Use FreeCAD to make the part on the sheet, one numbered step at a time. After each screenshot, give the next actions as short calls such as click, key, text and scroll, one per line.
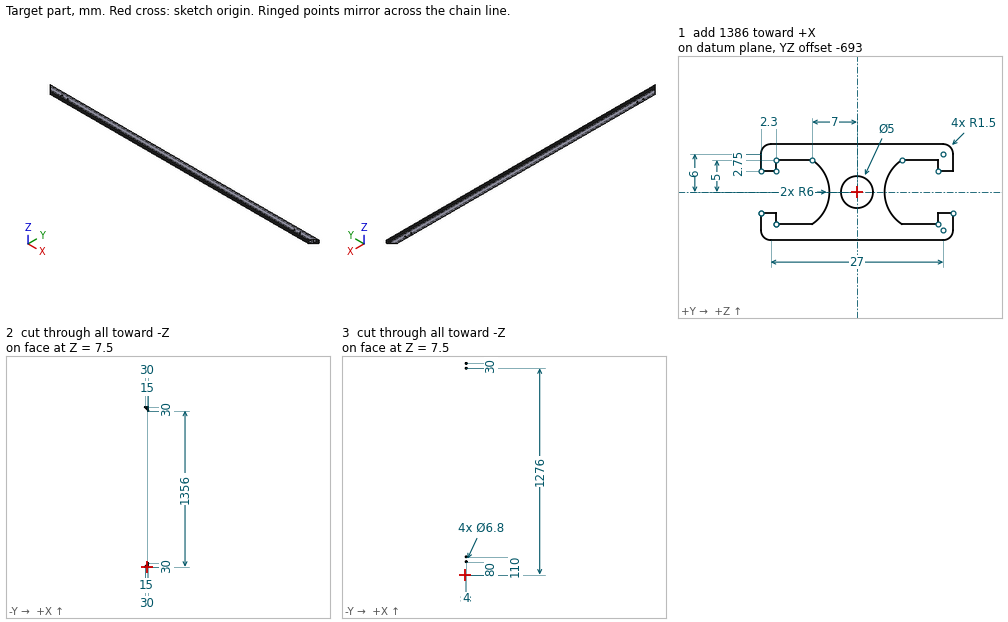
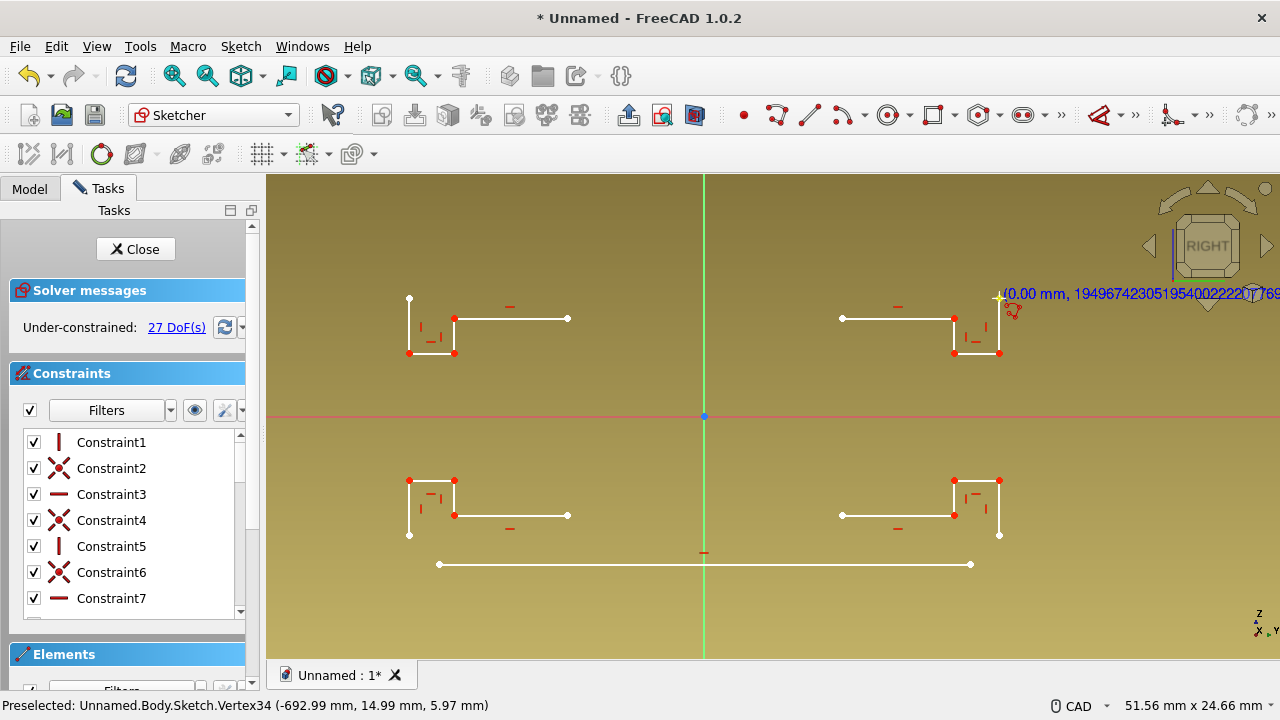
click(810, 116)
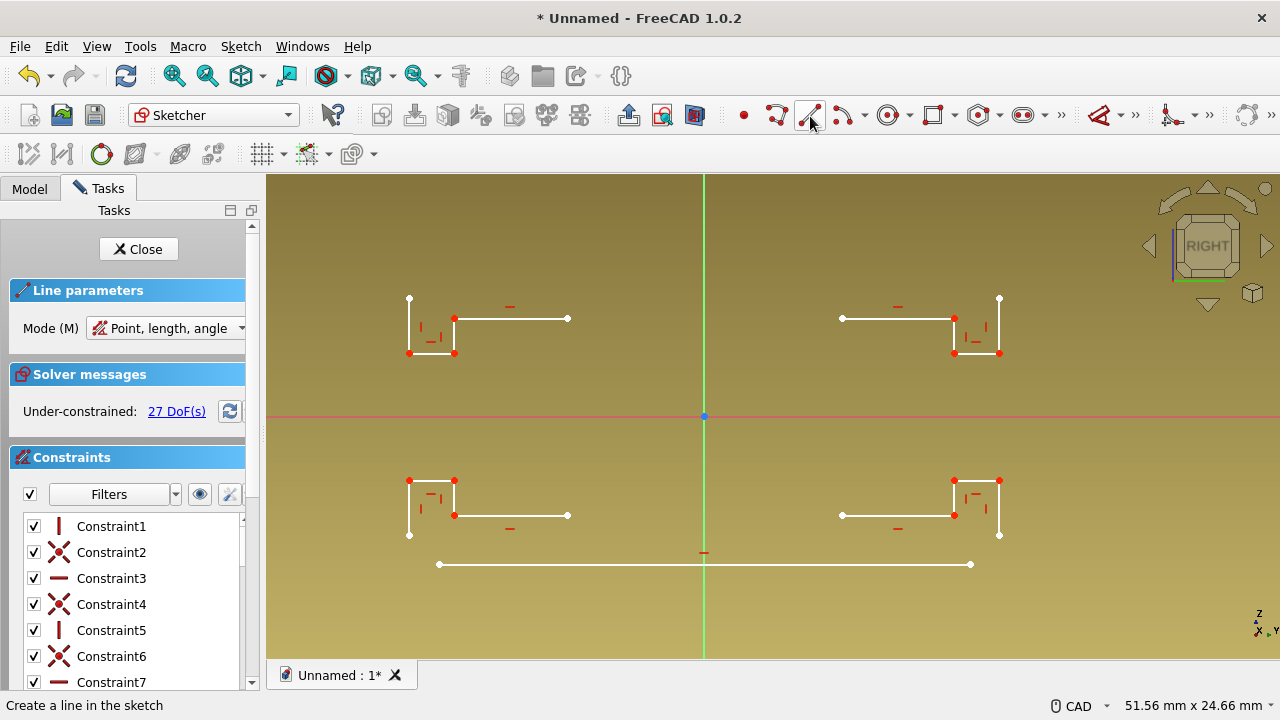
click(970, 269)
click(439, 269)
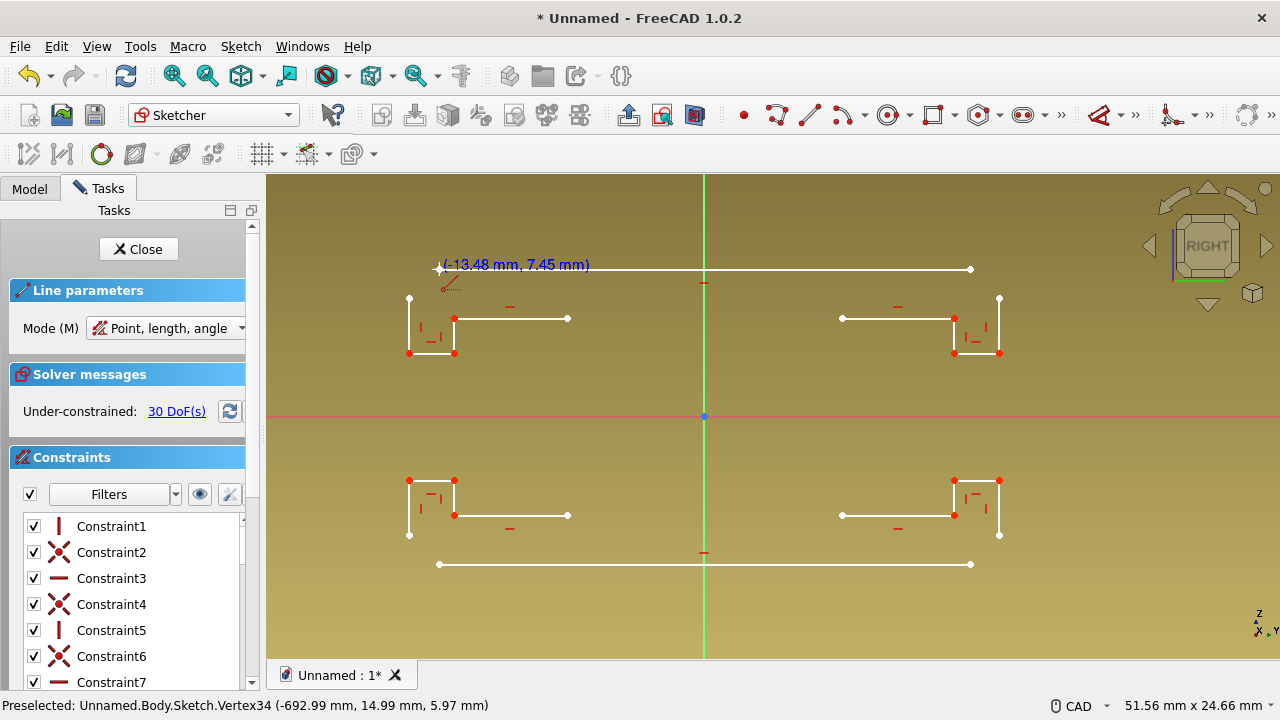
click(864, 116)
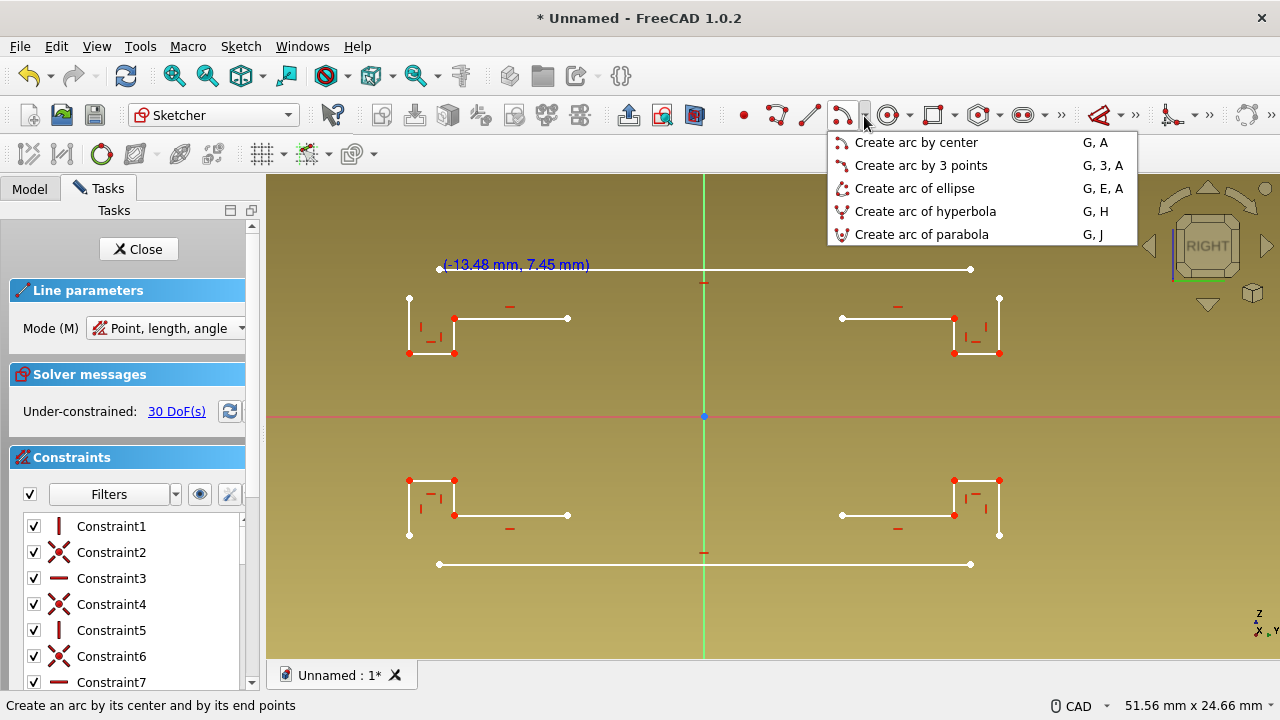
click(982, 166)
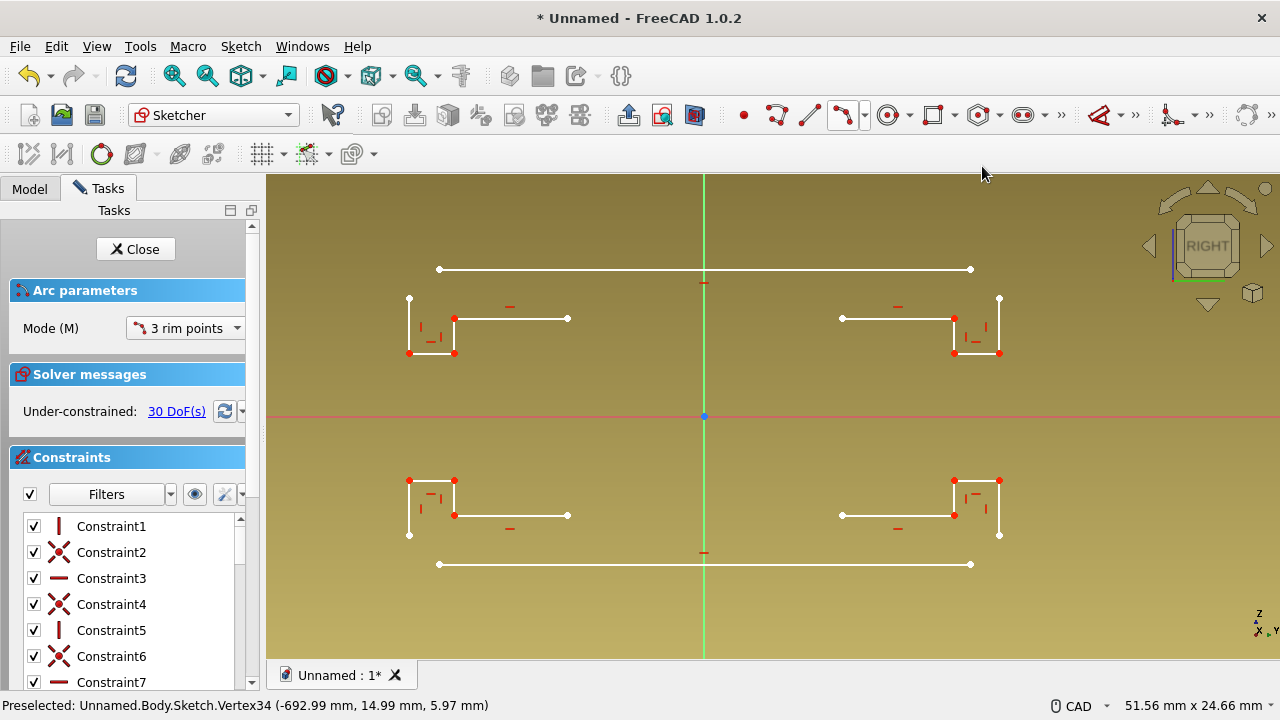
click(567, 319)
click(567, 516)
click(617, 440)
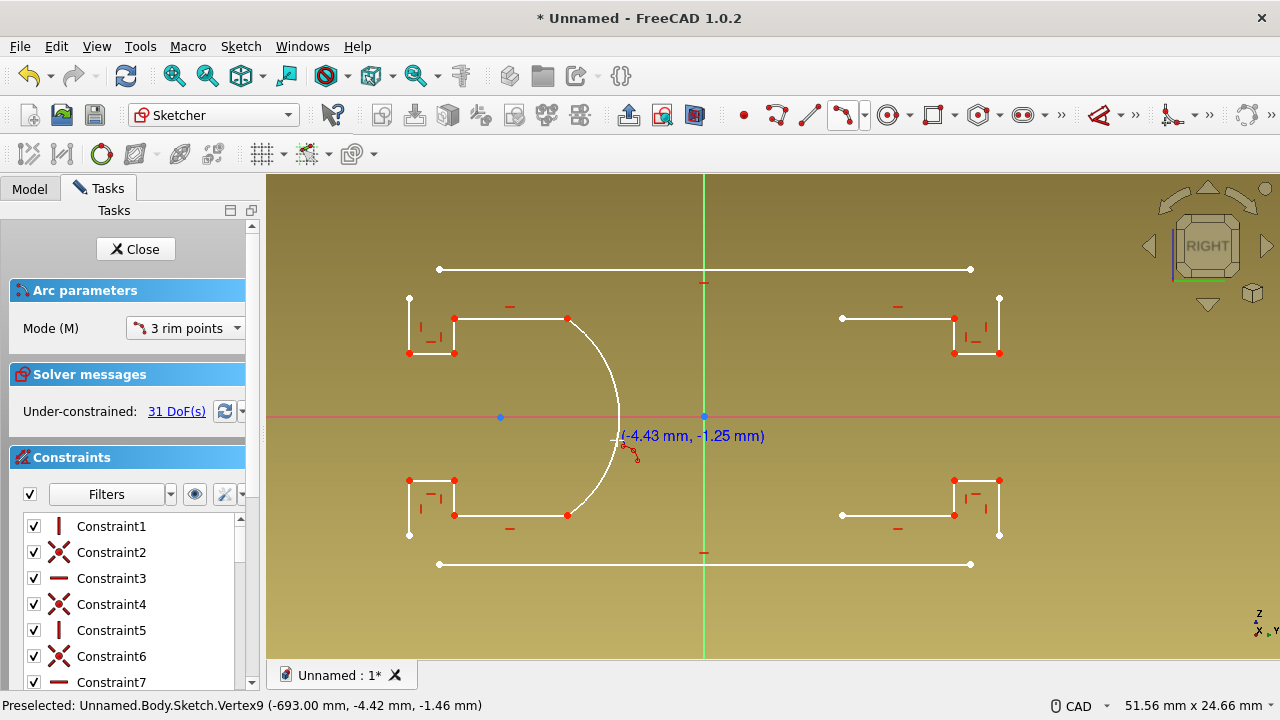
click(409, 536)
click(439, 565)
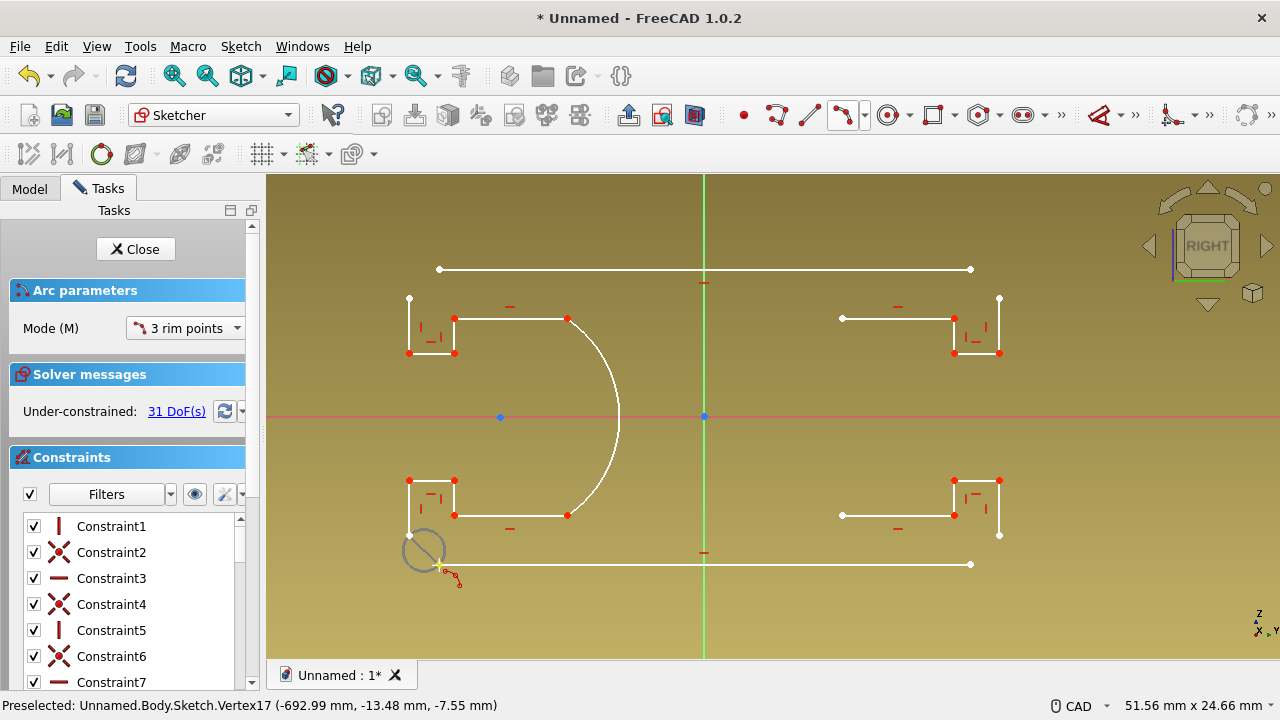
scroll(418, 555, up, 4)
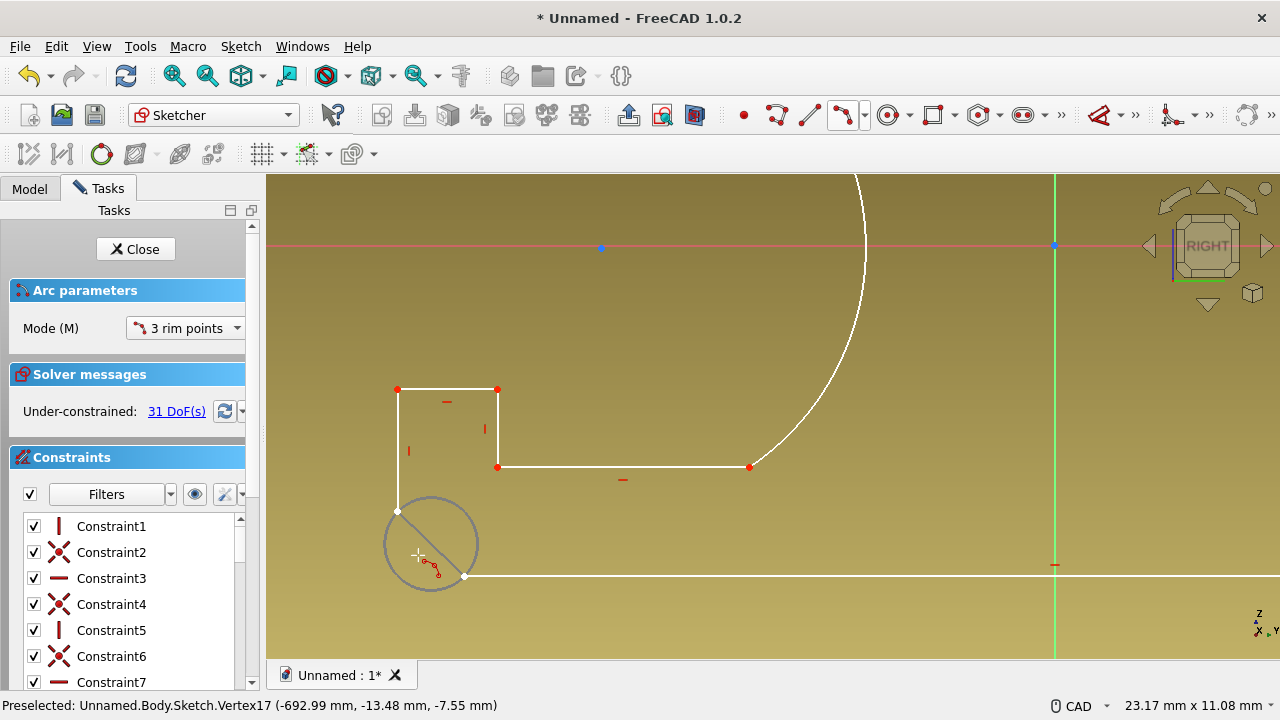
click(417, 555)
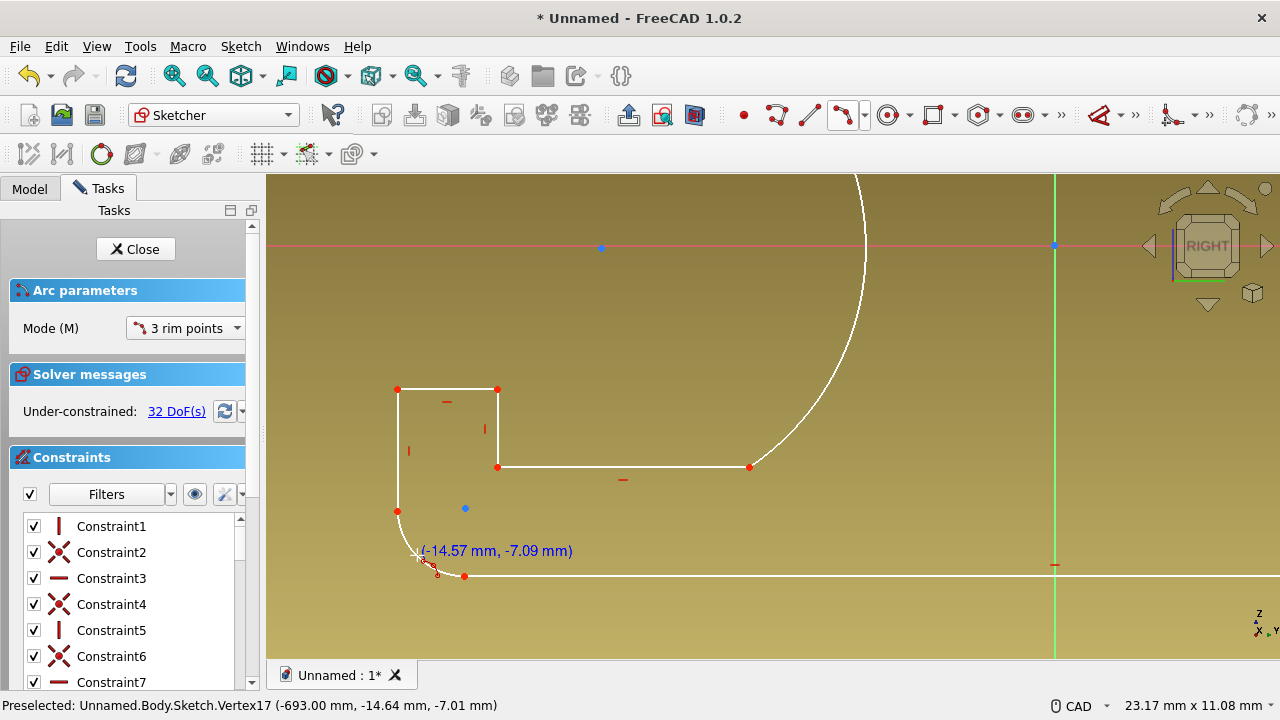
scroll(419, 556, down, 4)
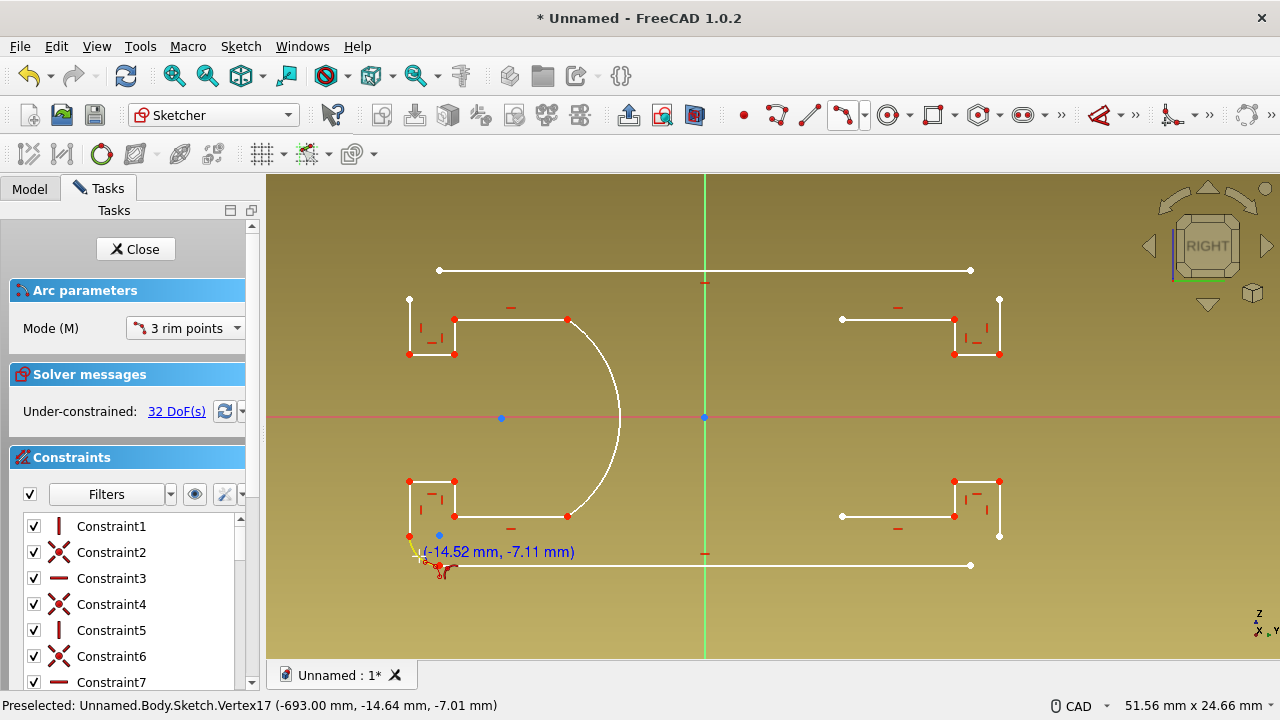
click(971, 566)
click(1000, 537)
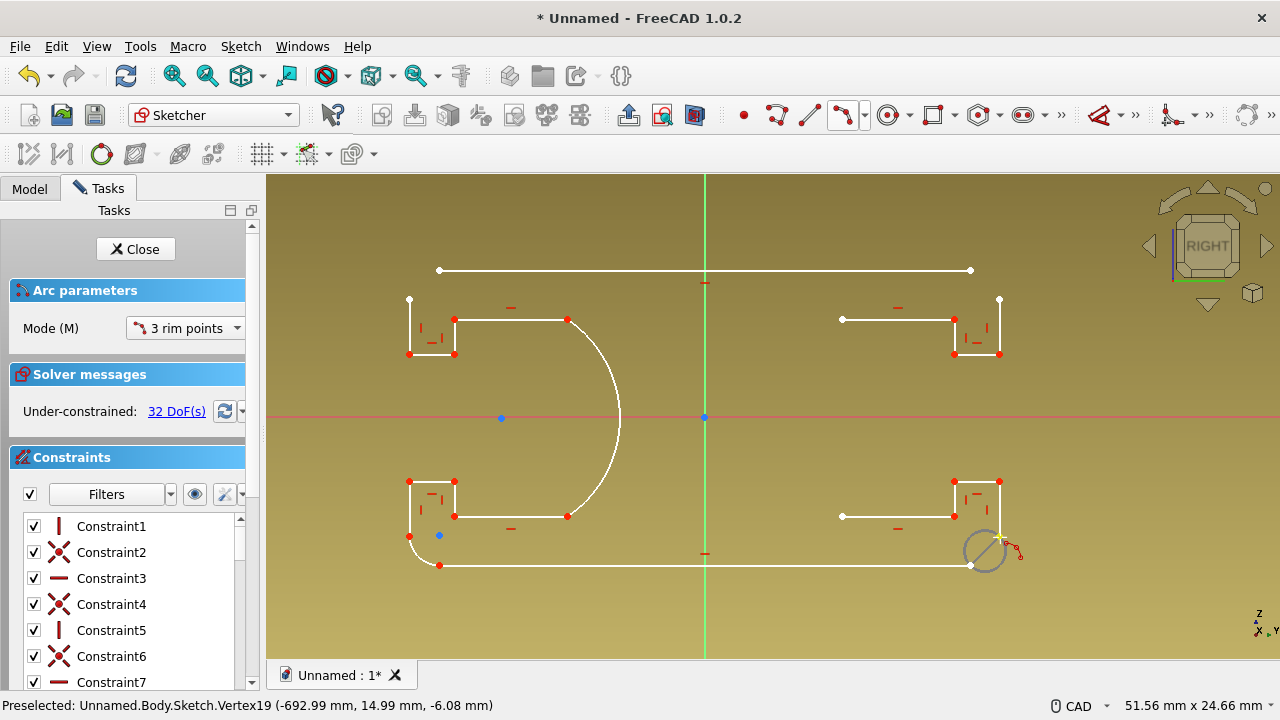
scroll(991, 556, up, 4)